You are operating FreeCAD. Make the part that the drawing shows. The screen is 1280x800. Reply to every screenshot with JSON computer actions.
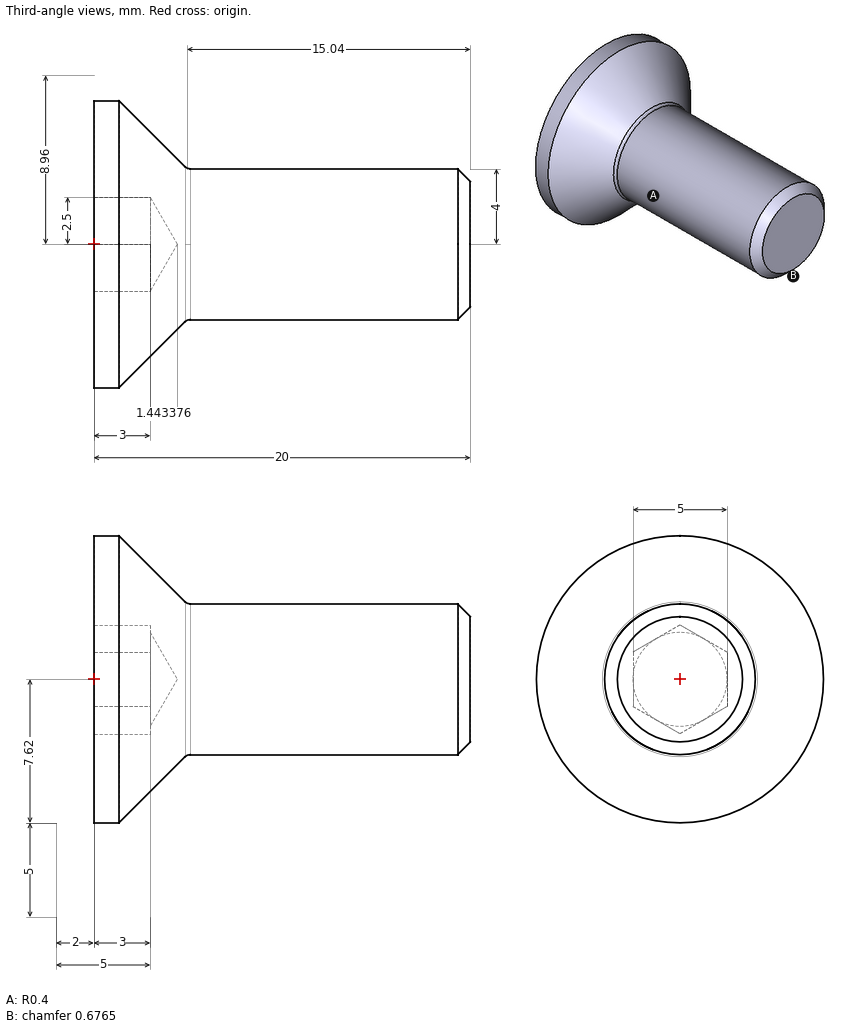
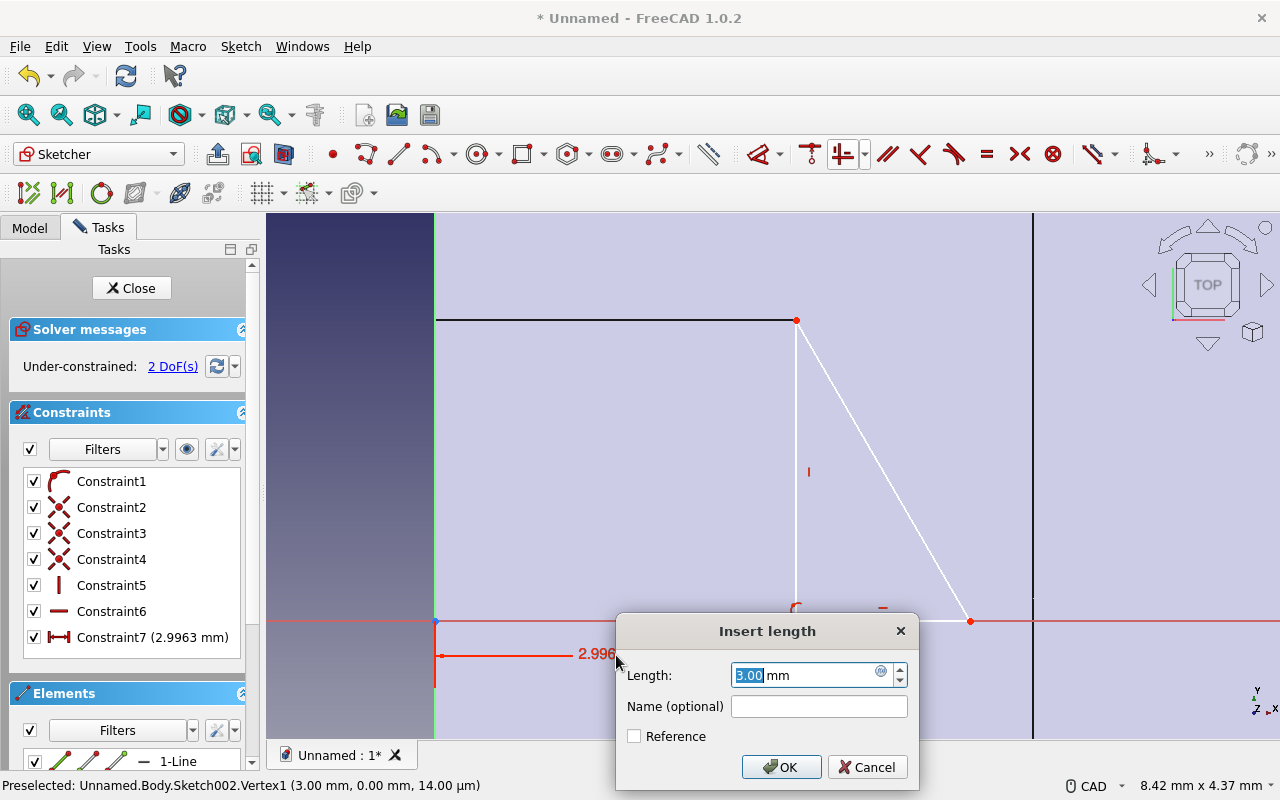
{"action": "type", "text": "3"}
{"action": "key", "text": "Return"}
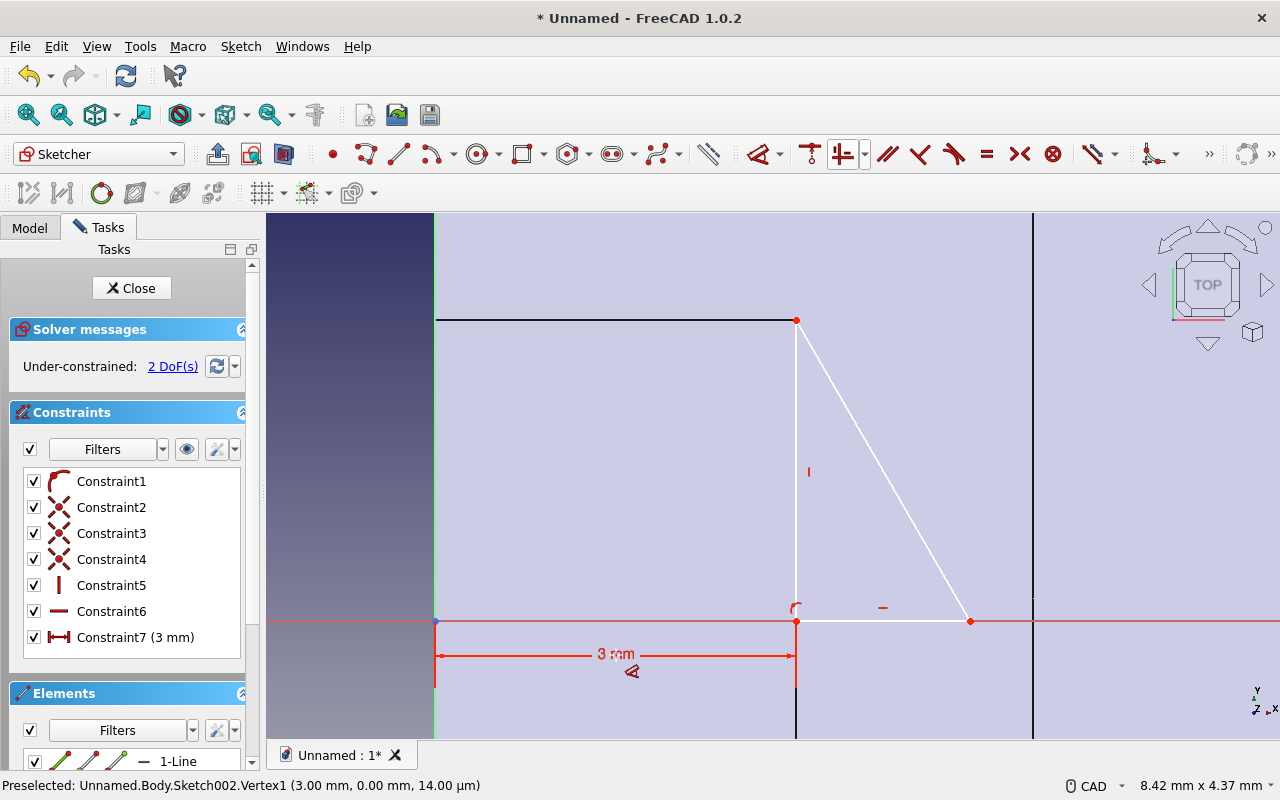
{"action": "left_click", "coordinate": [796, 411]}
{"action": "left_click", "coordinate": [830, 471]}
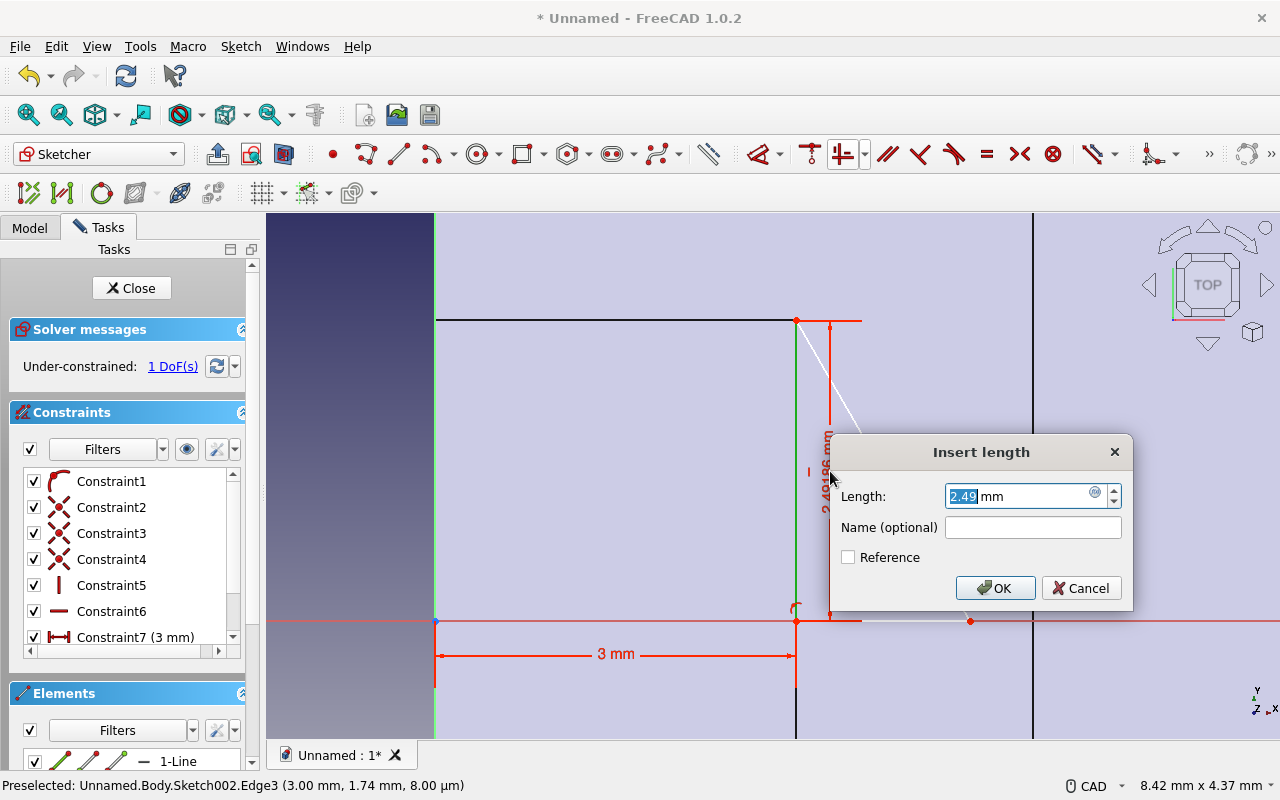
{"action": "type", "text": "2.5"}
{"action": "key", "text": "Return"}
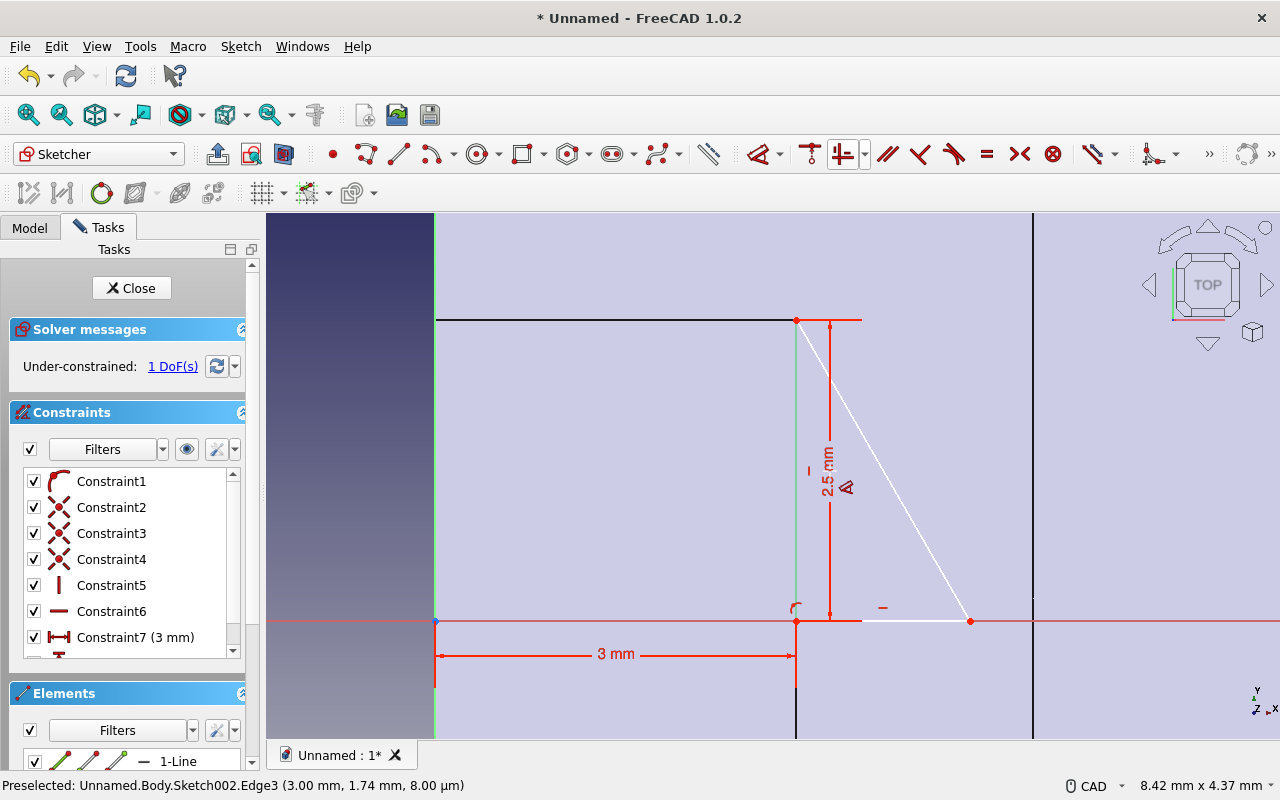
{"action": "left_click", "coordinate": [849, 621]}
{"action": "left_click", "coordinate": [883, 655]}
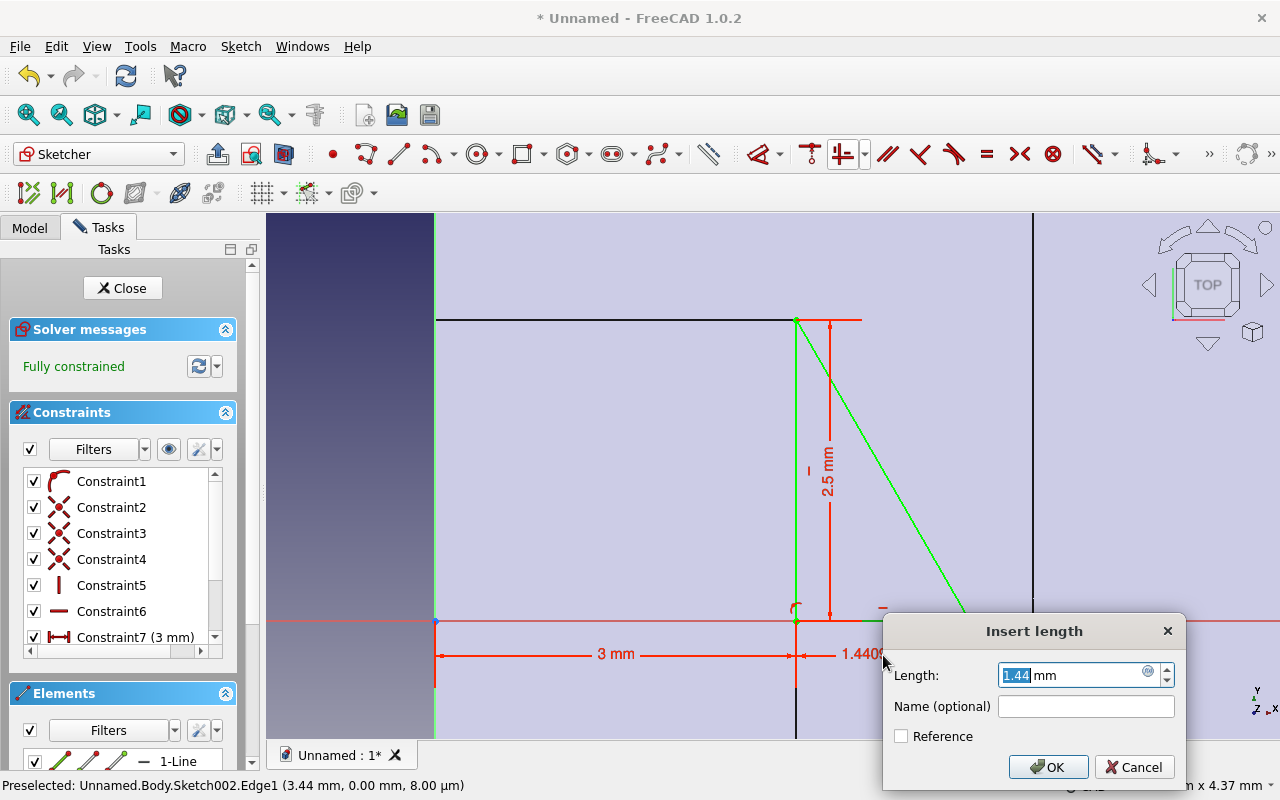
{"action": "type", "text": "1.443376"}
{"action": "key", "text": "Return"}
{"action": "key", "text": "Escape"}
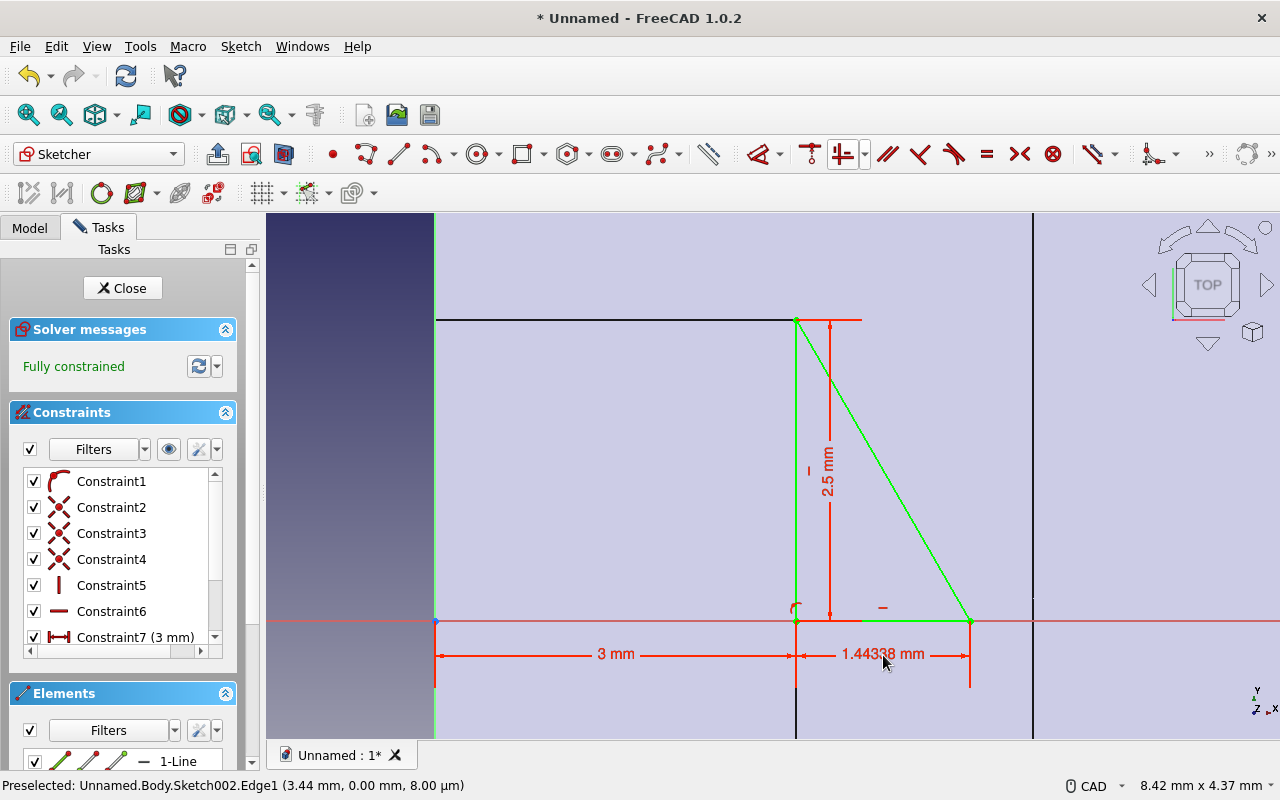
{"action": "left_click", "coordinate": [123, 288]}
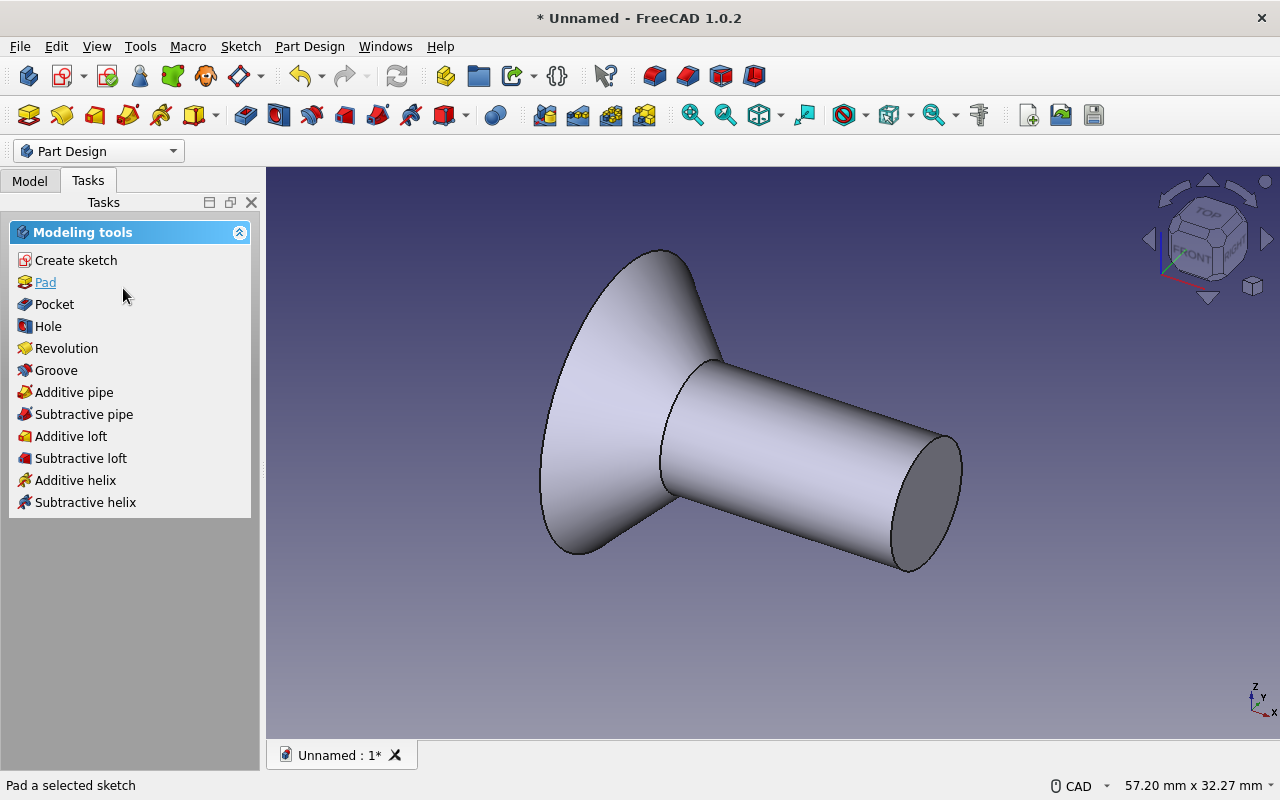
{"action": "left_click", "coordinate": [312, 116]}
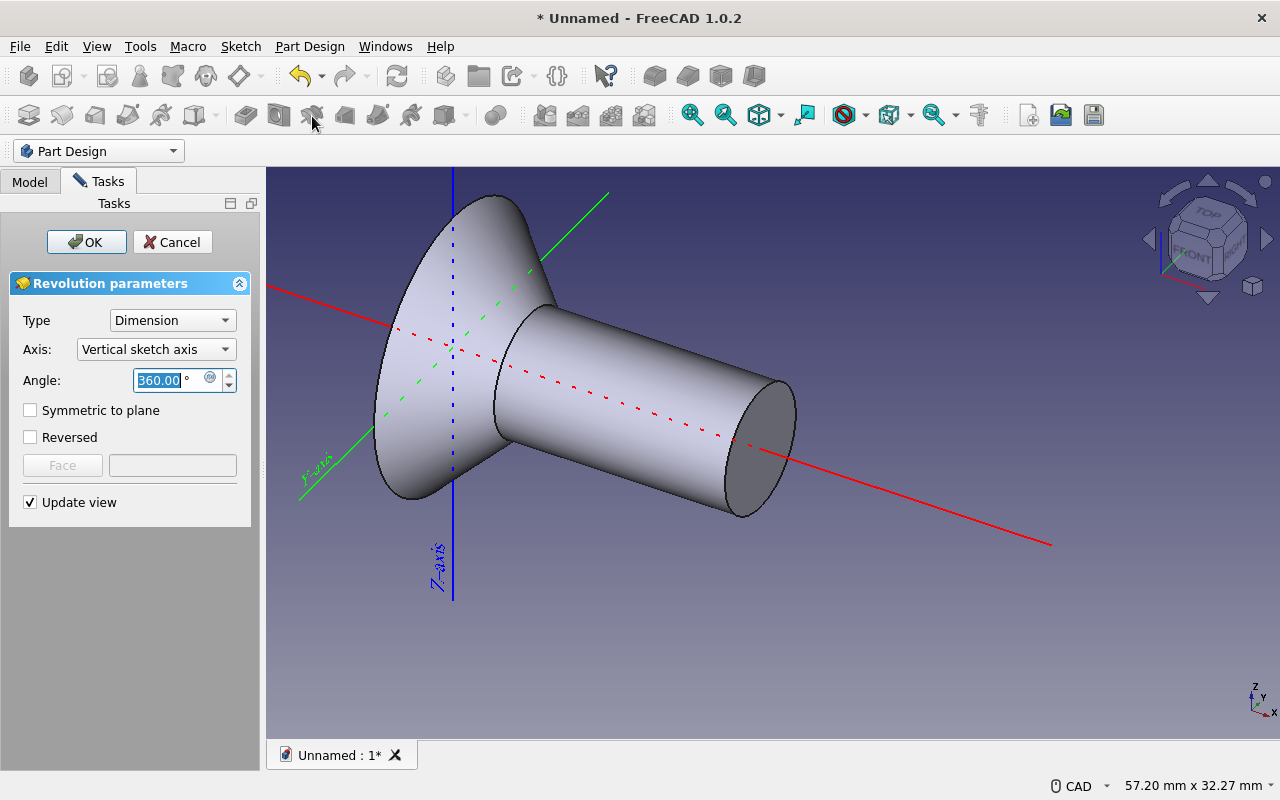
{"action": "left_click", "coordinate": [157, 350]}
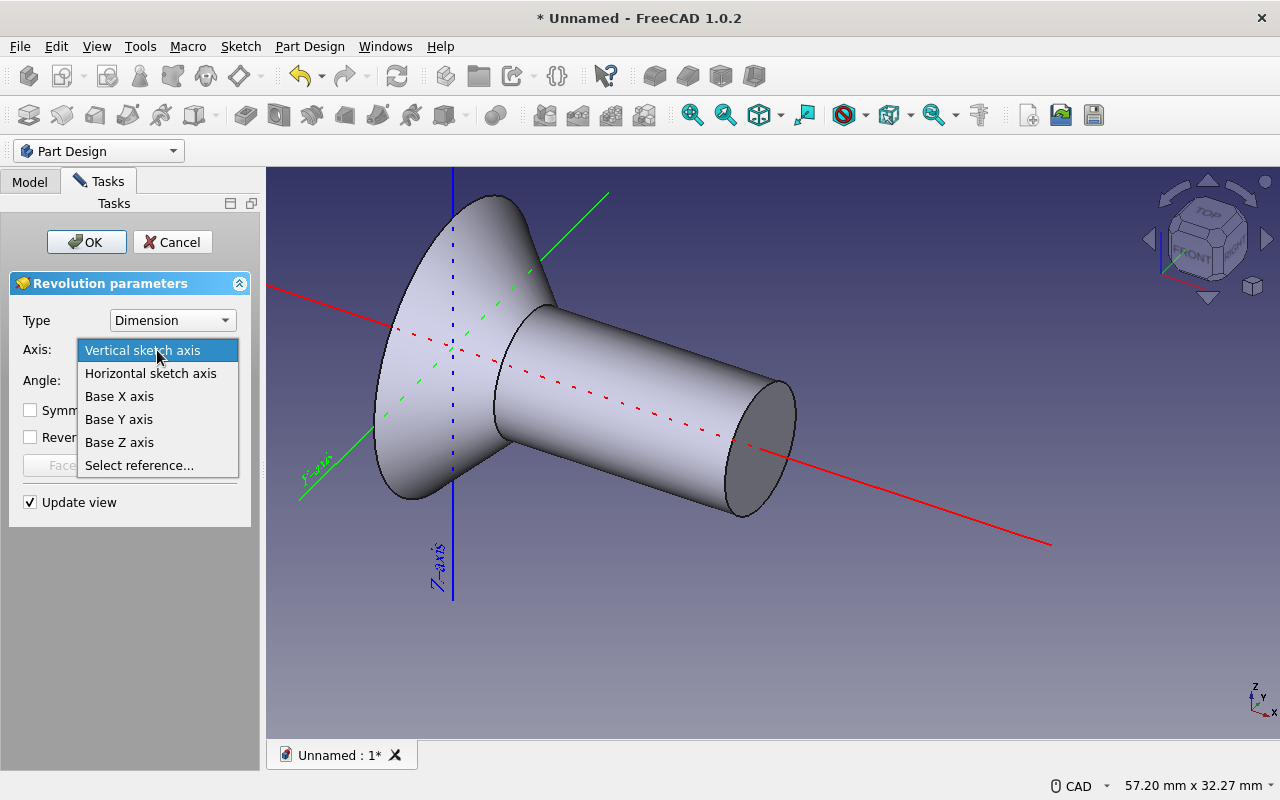
{"action": "left_click", "coordinate": [156, 374]}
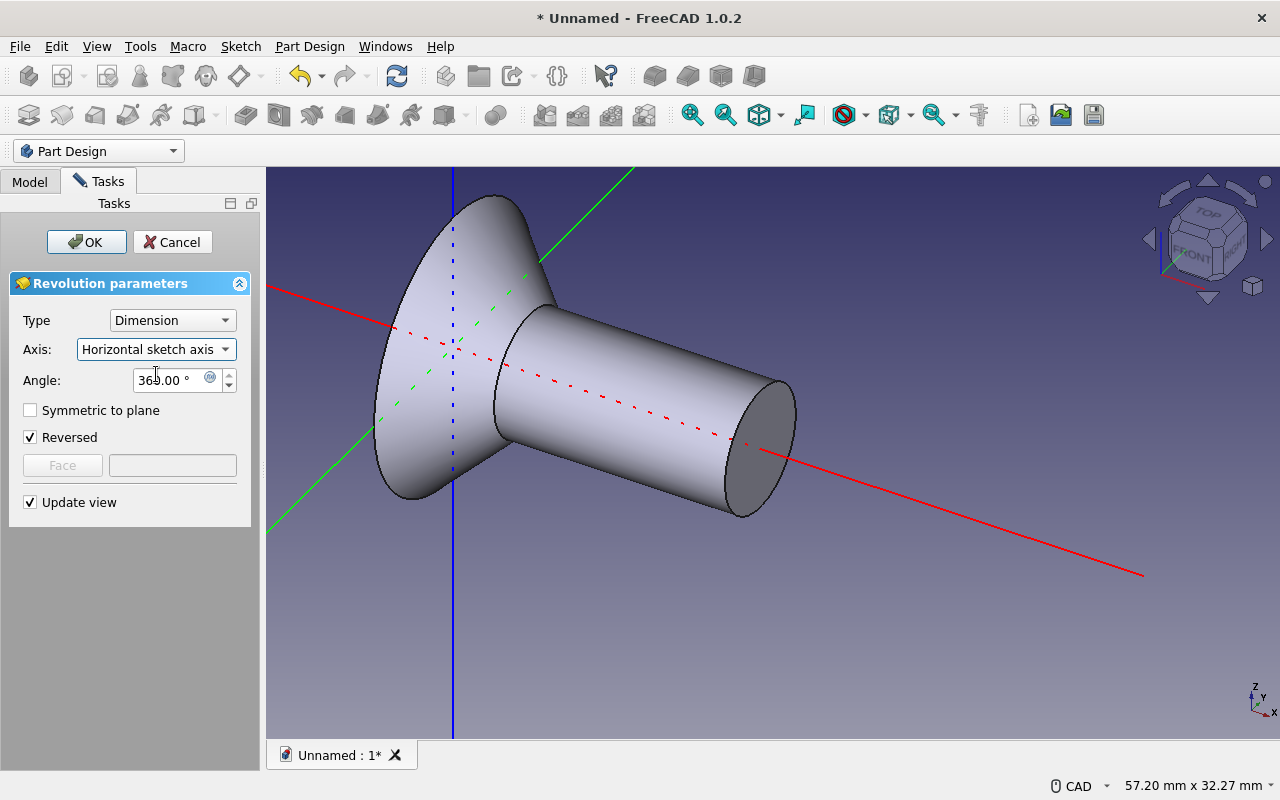
{"action": "left_click", "coordinate": [87, 242]}